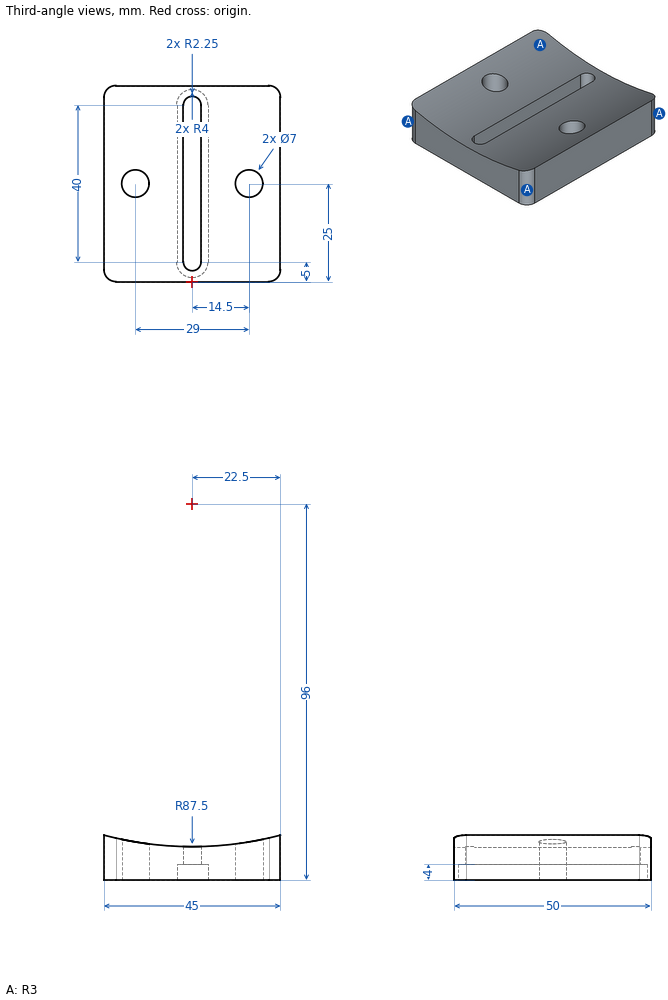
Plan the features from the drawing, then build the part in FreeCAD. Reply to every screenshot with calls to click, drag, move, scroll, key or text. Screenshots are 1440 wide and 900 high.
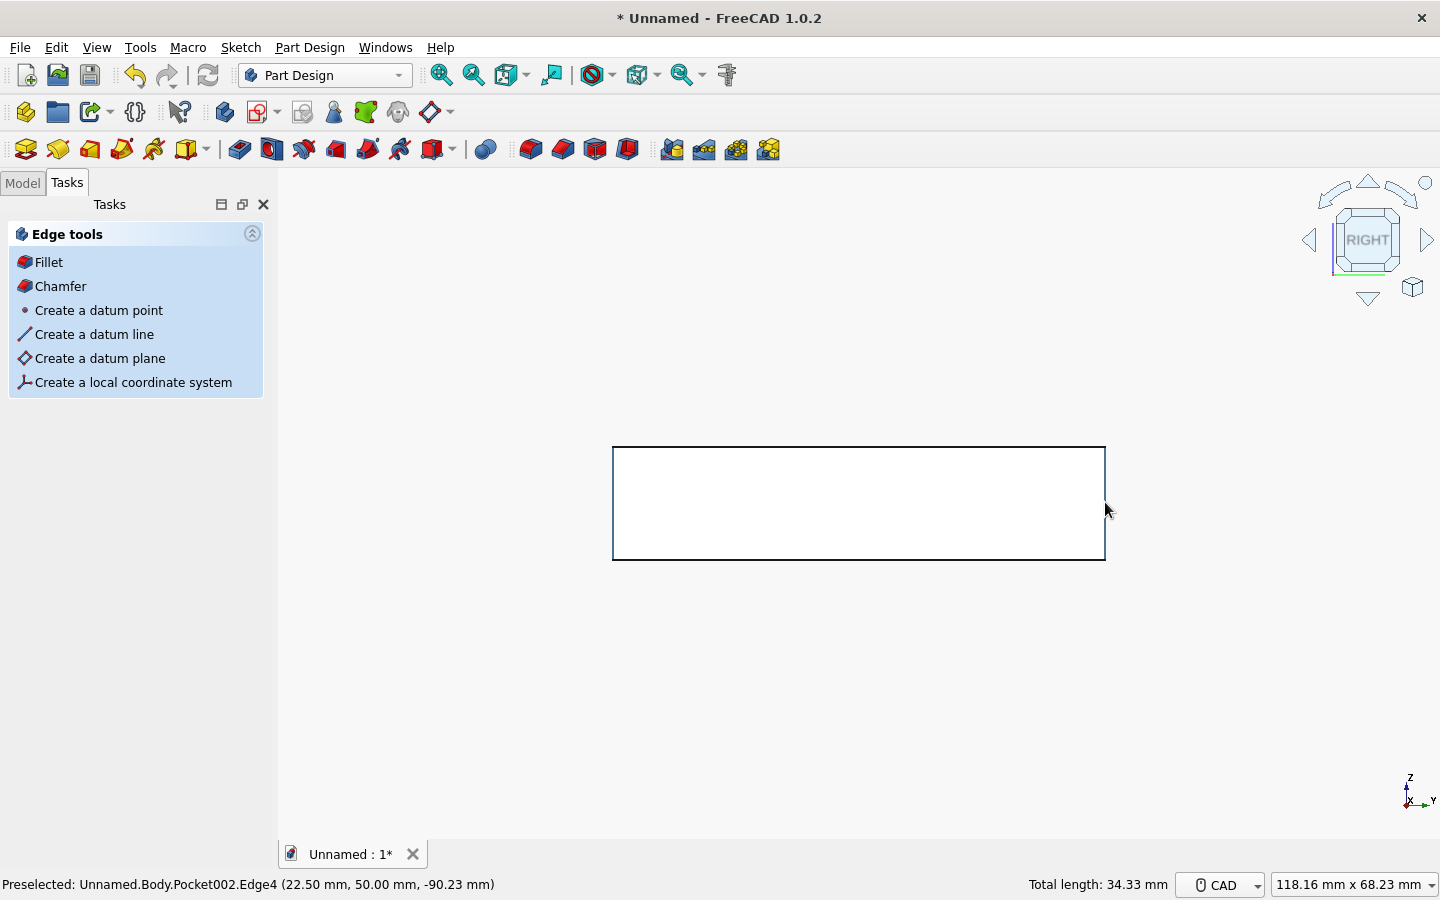
key(5)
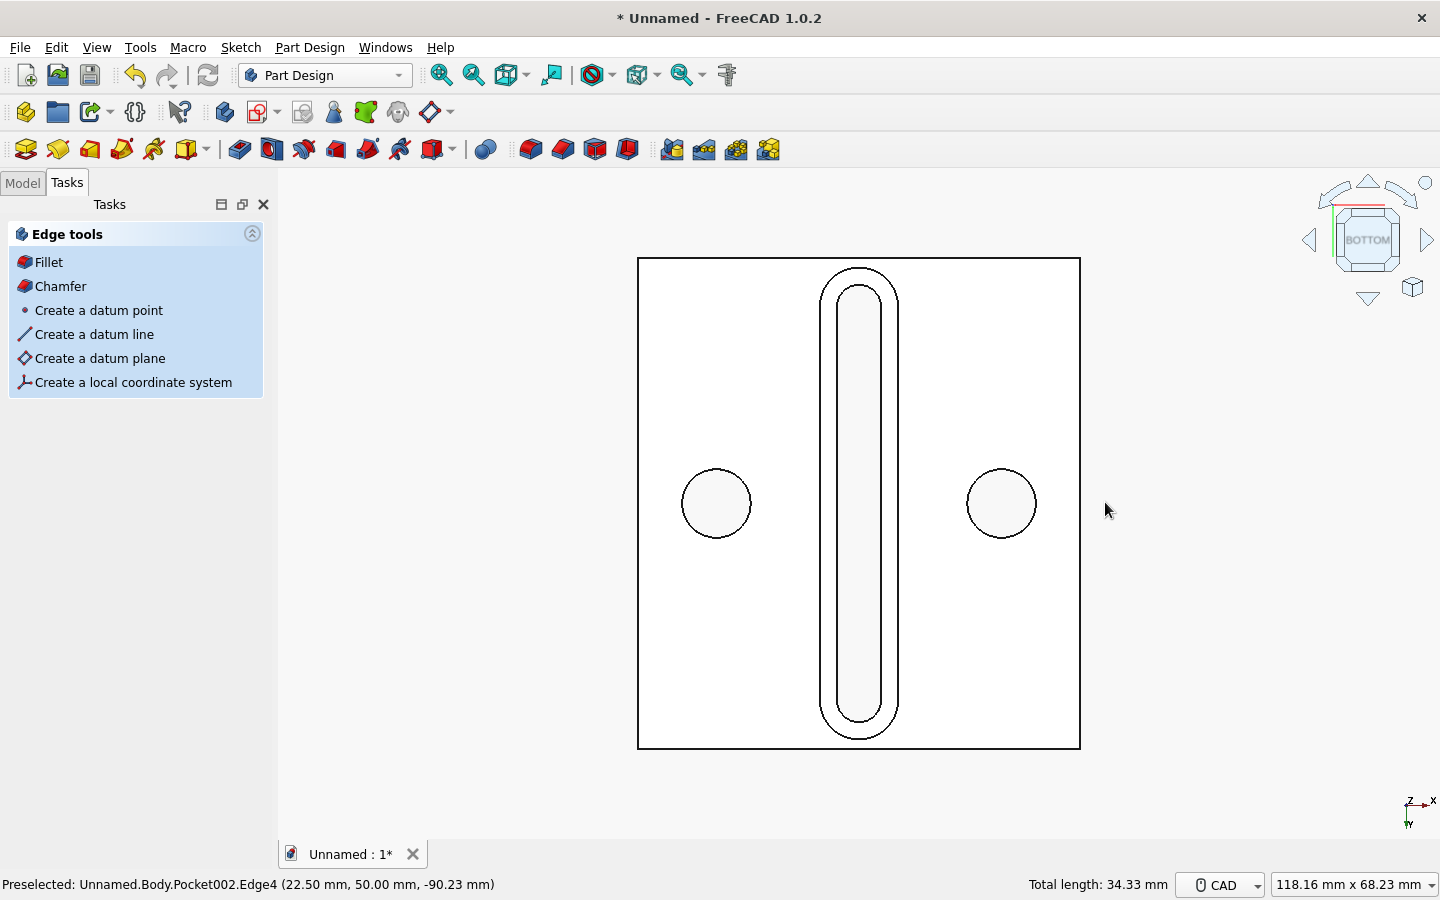
key(4)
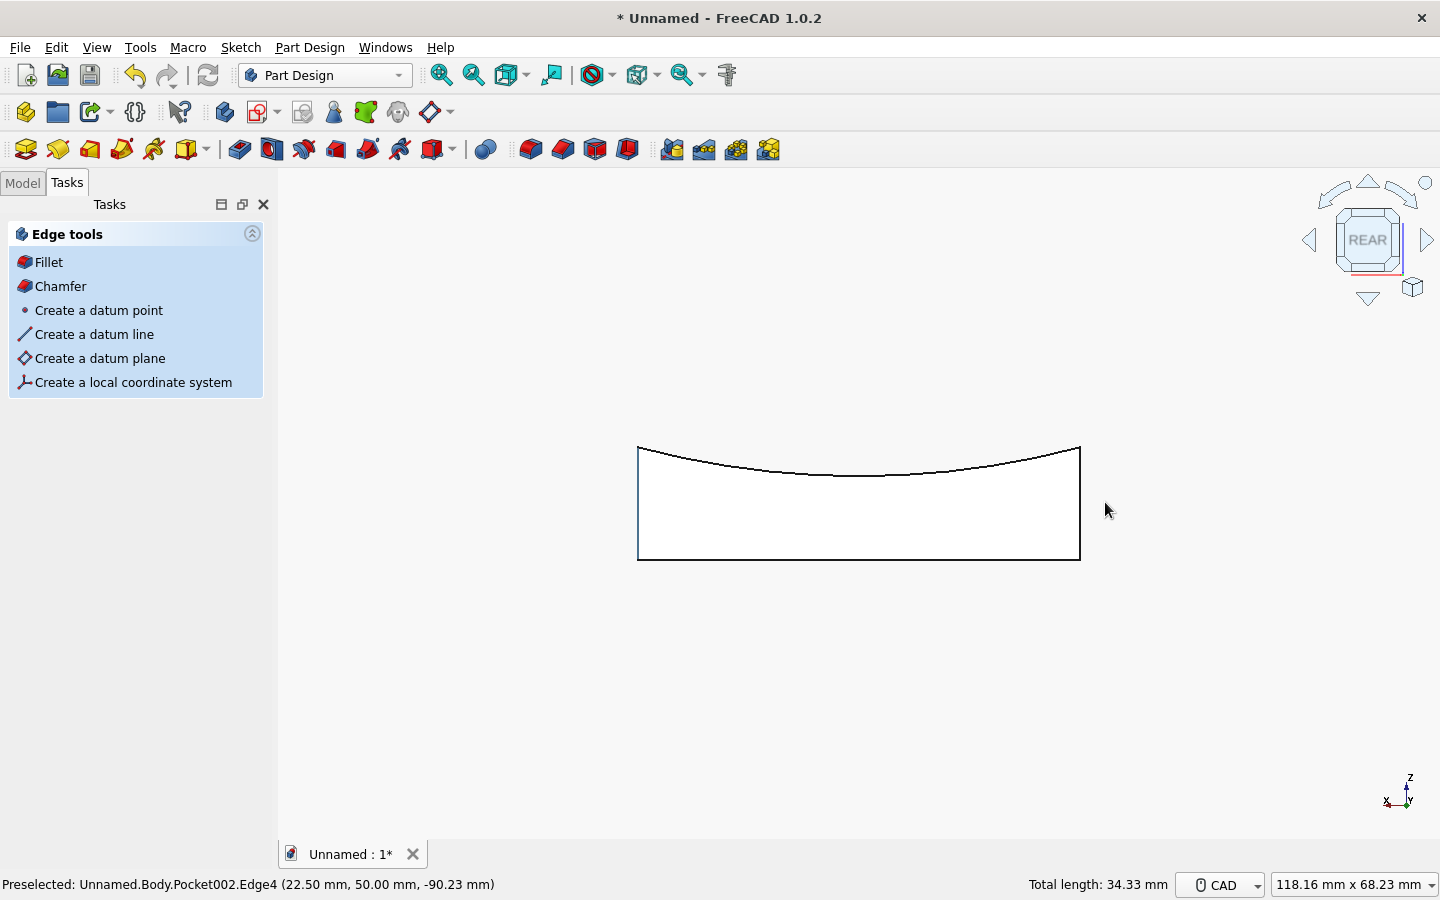
click(442, 76)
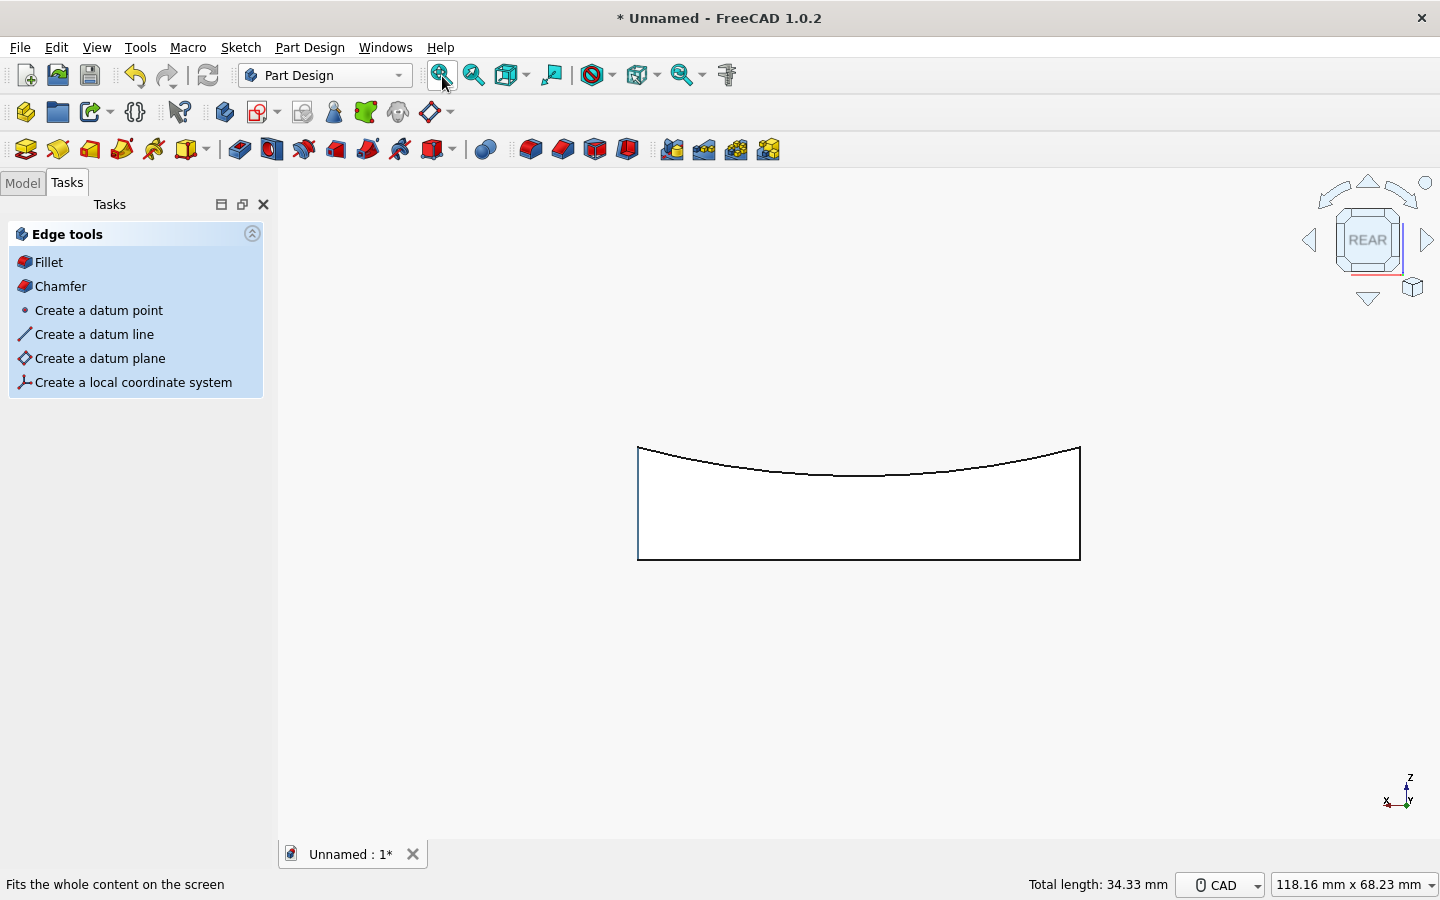
click(1080, 502, ctrl)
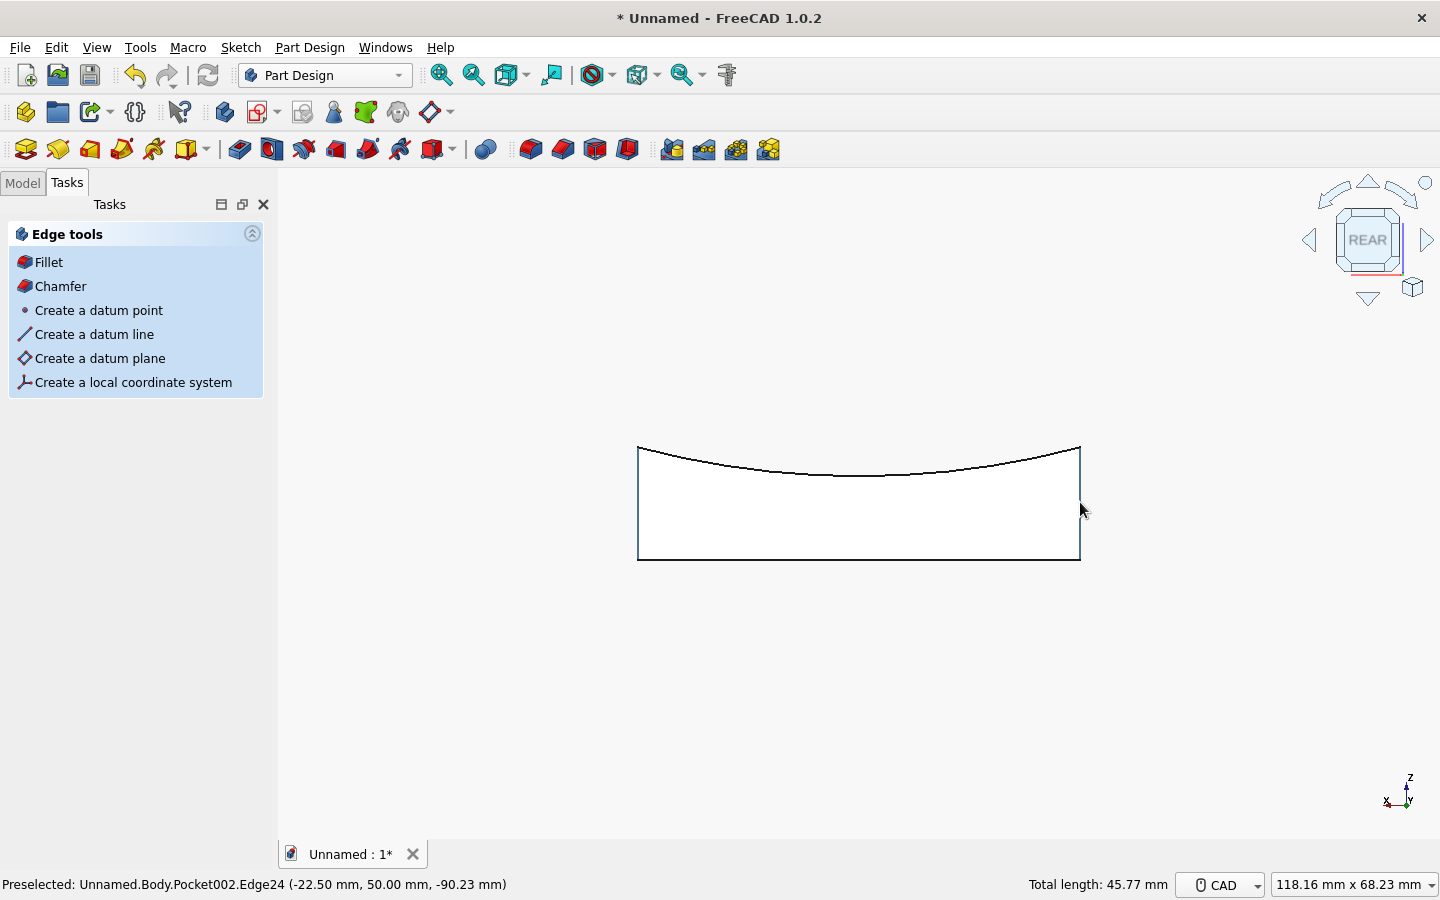
click(532, 150)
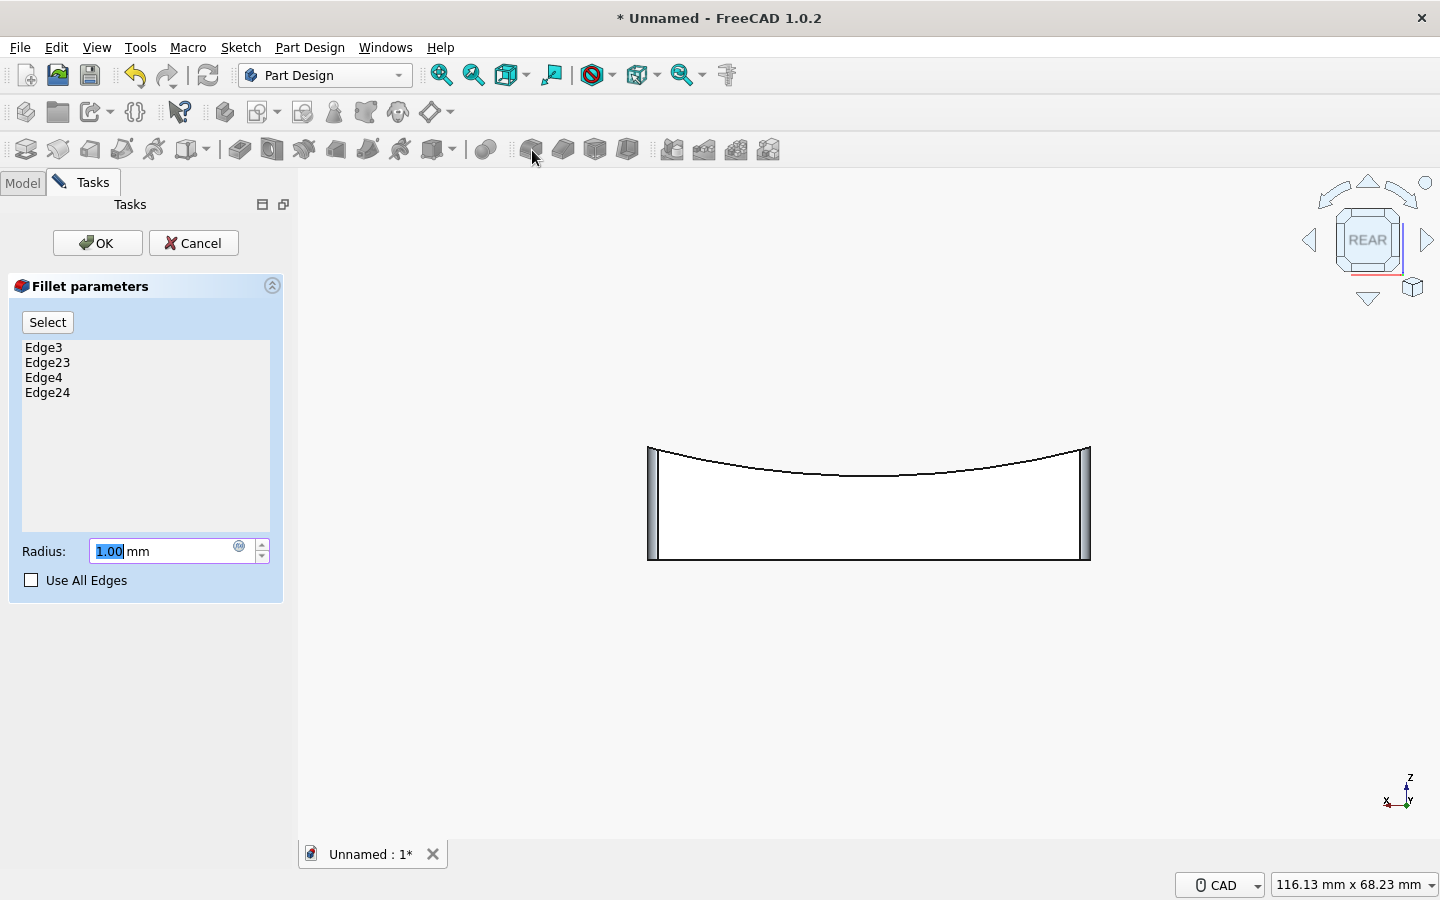
text(3)
key(Tab)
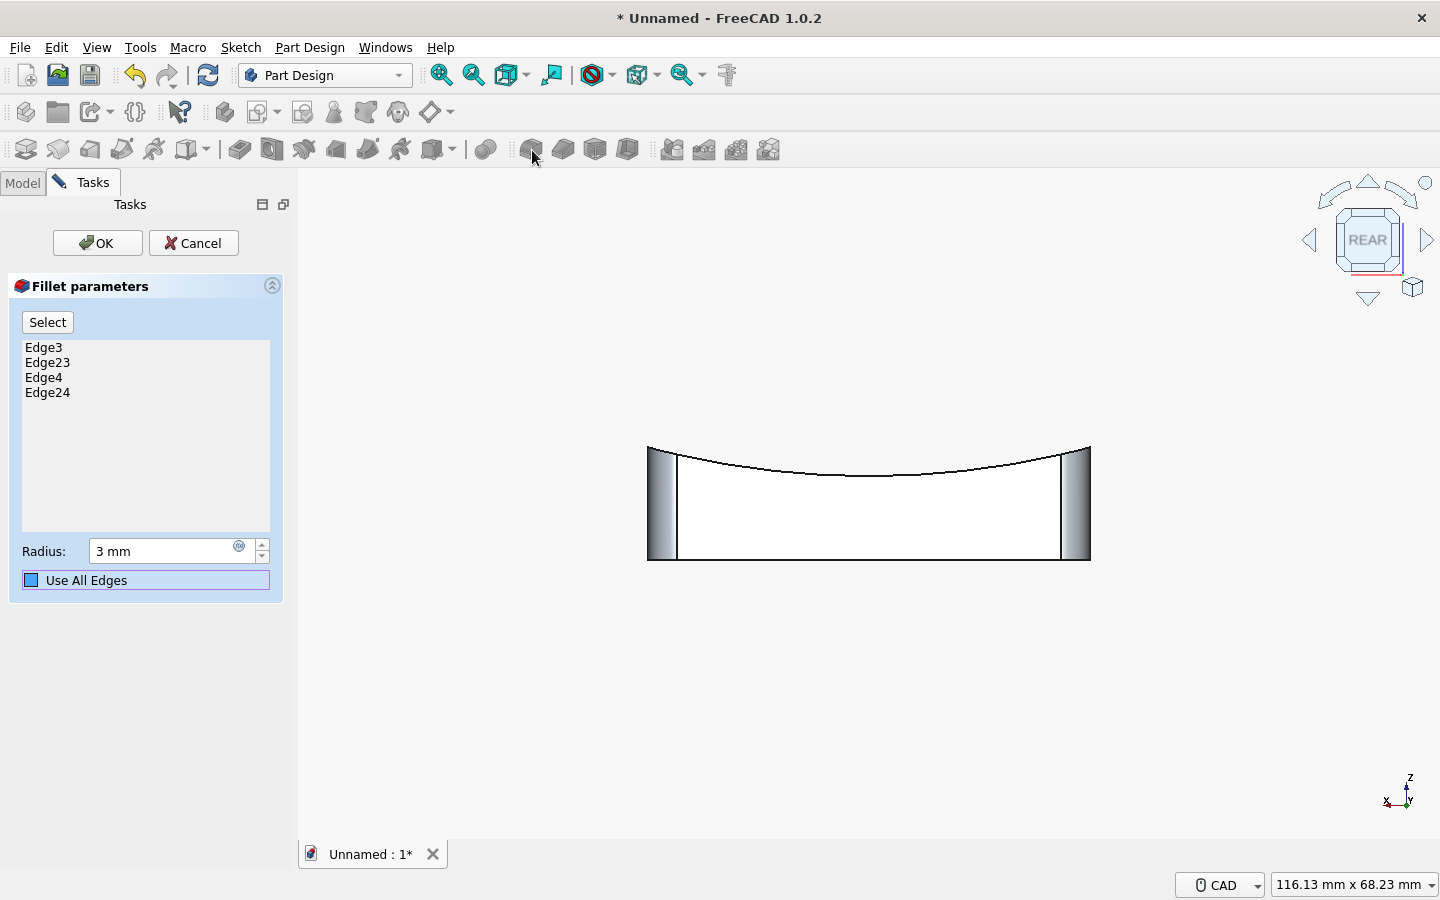
click(98, 243)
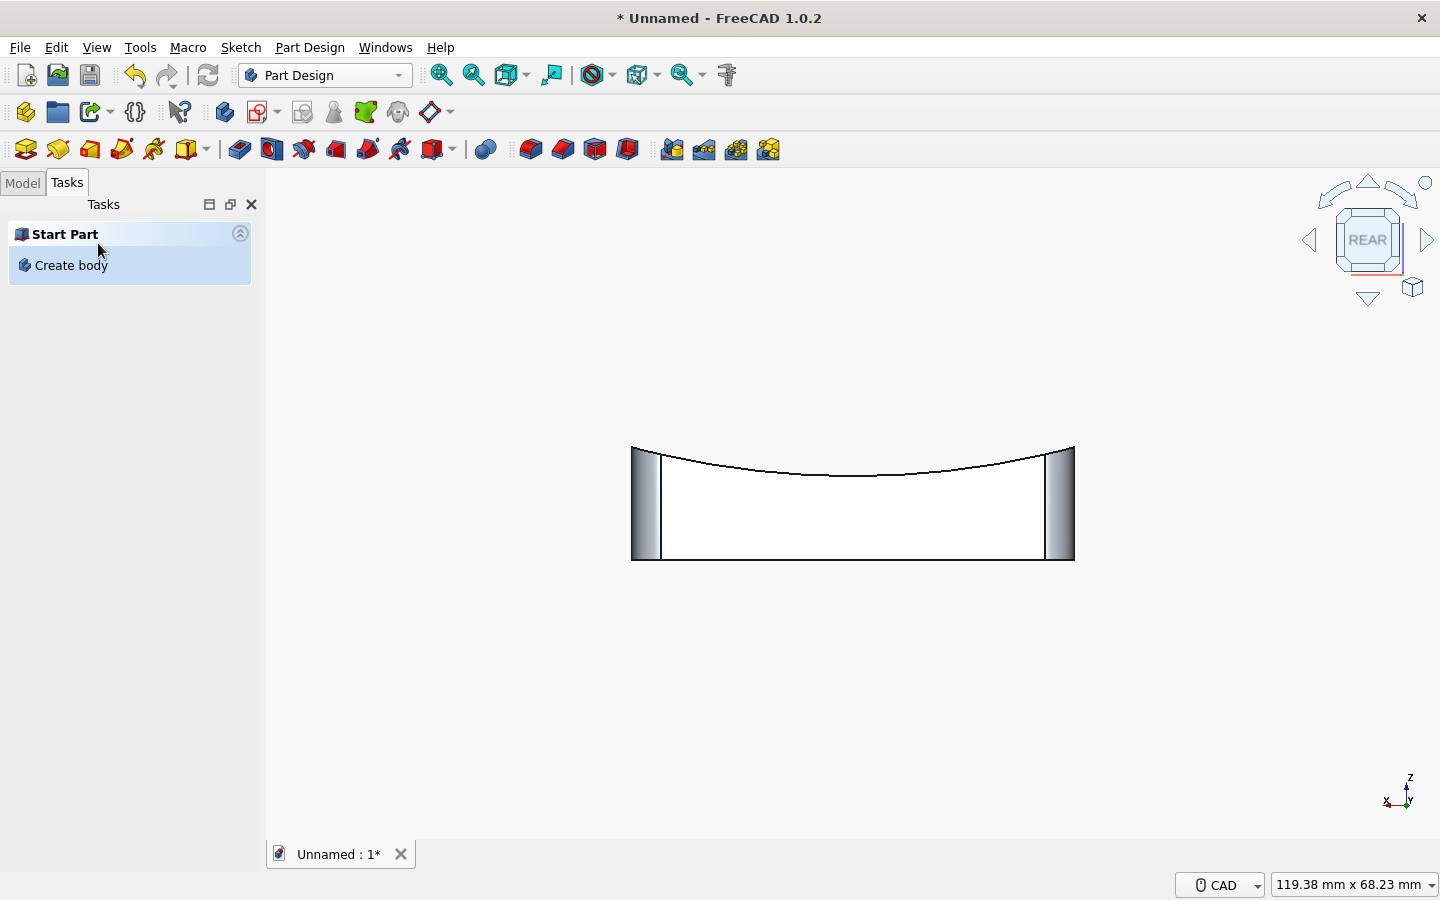
key(0)